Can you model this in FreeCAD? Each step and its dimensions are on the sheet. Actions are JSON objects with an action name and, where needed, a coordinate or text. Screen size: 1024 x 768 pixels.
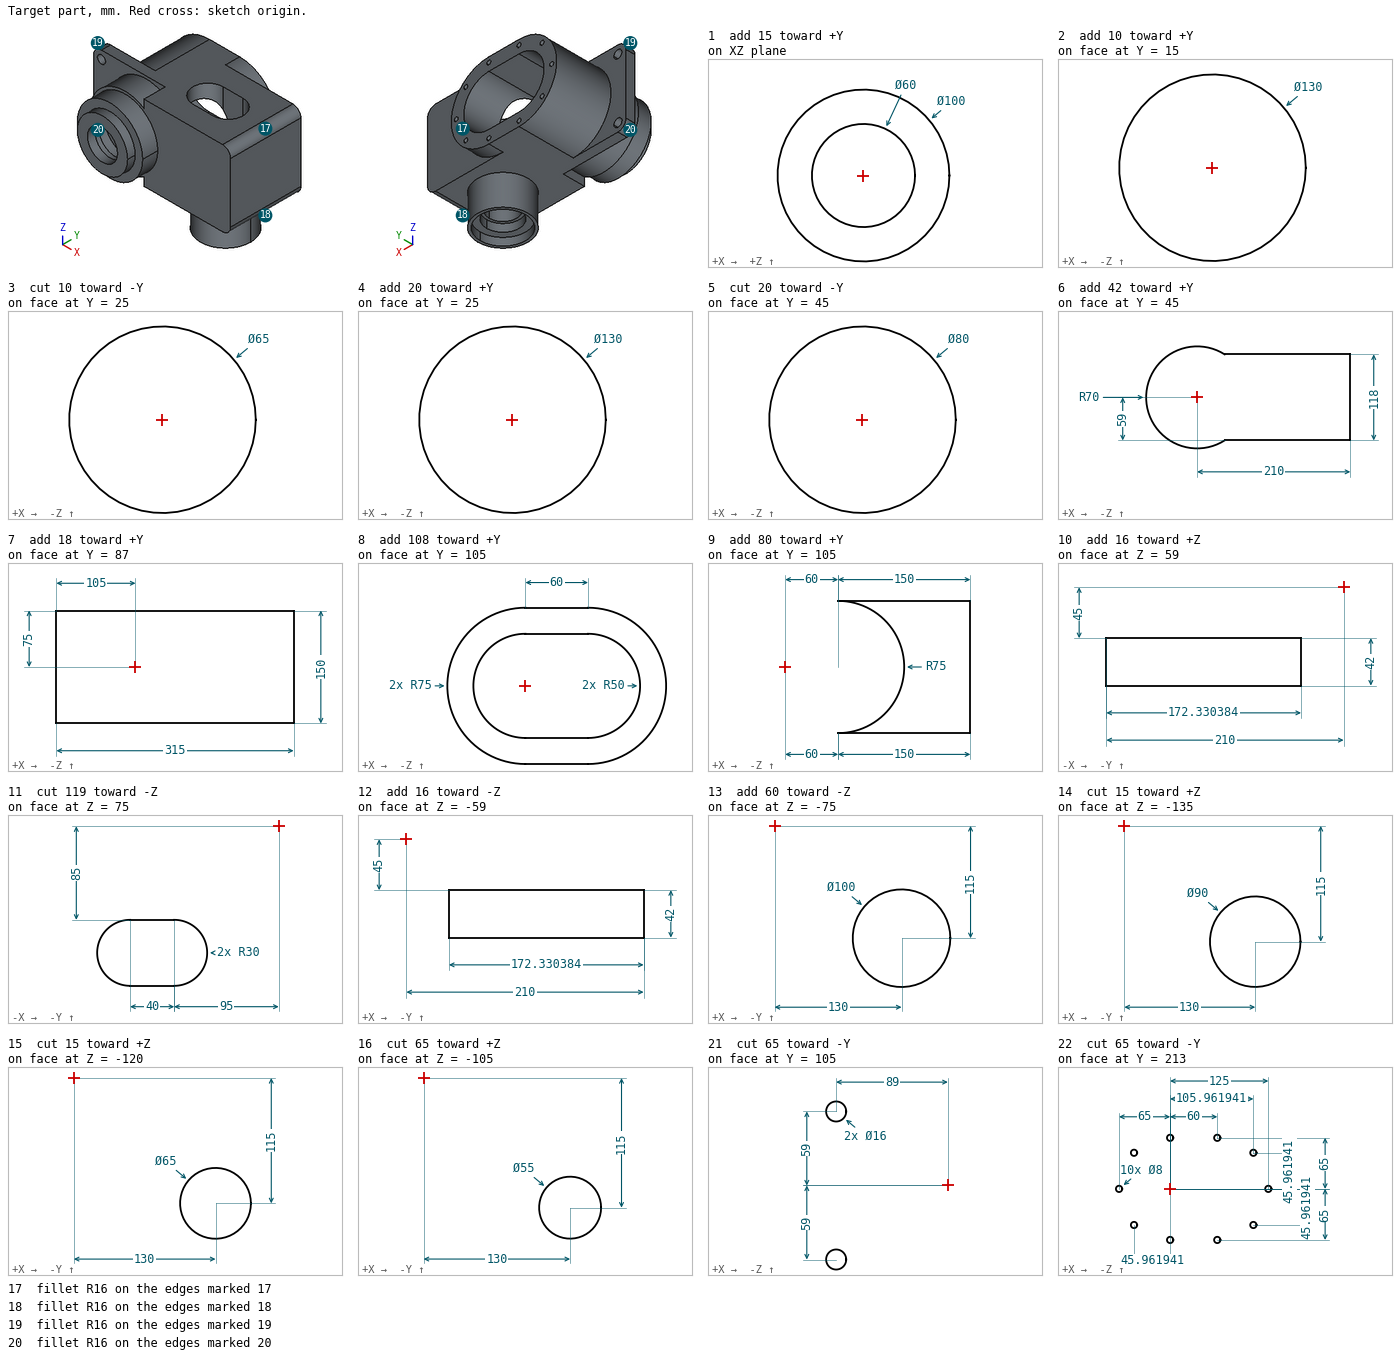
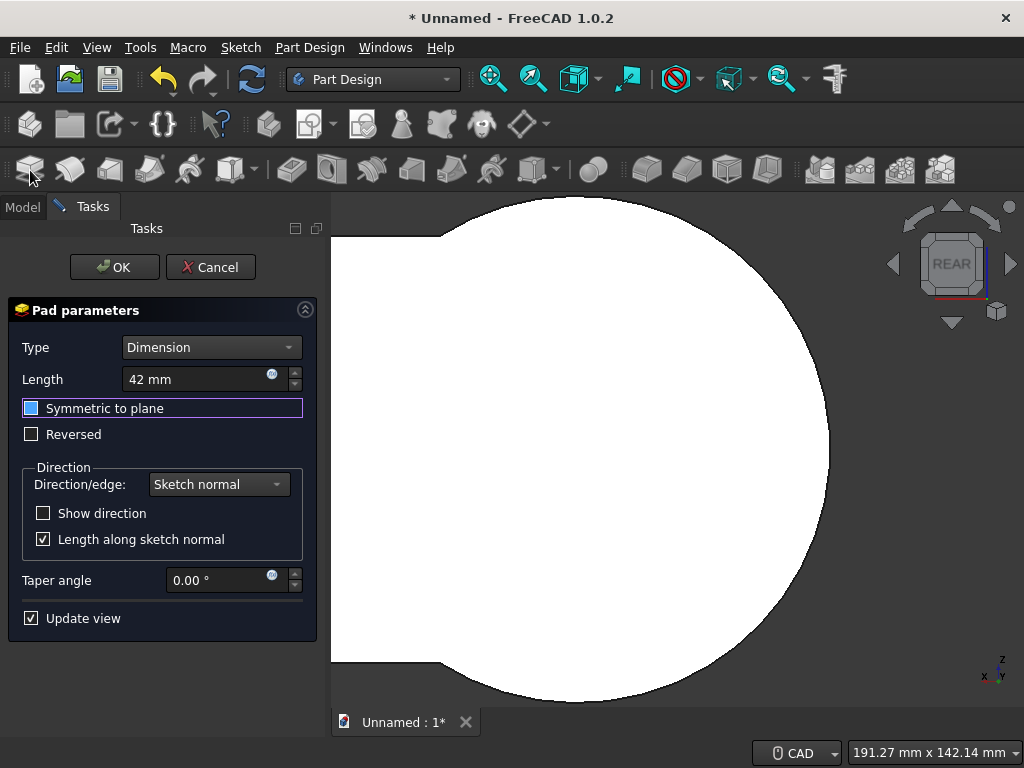
{"action": "left_click", "coordinate": [115, 267]}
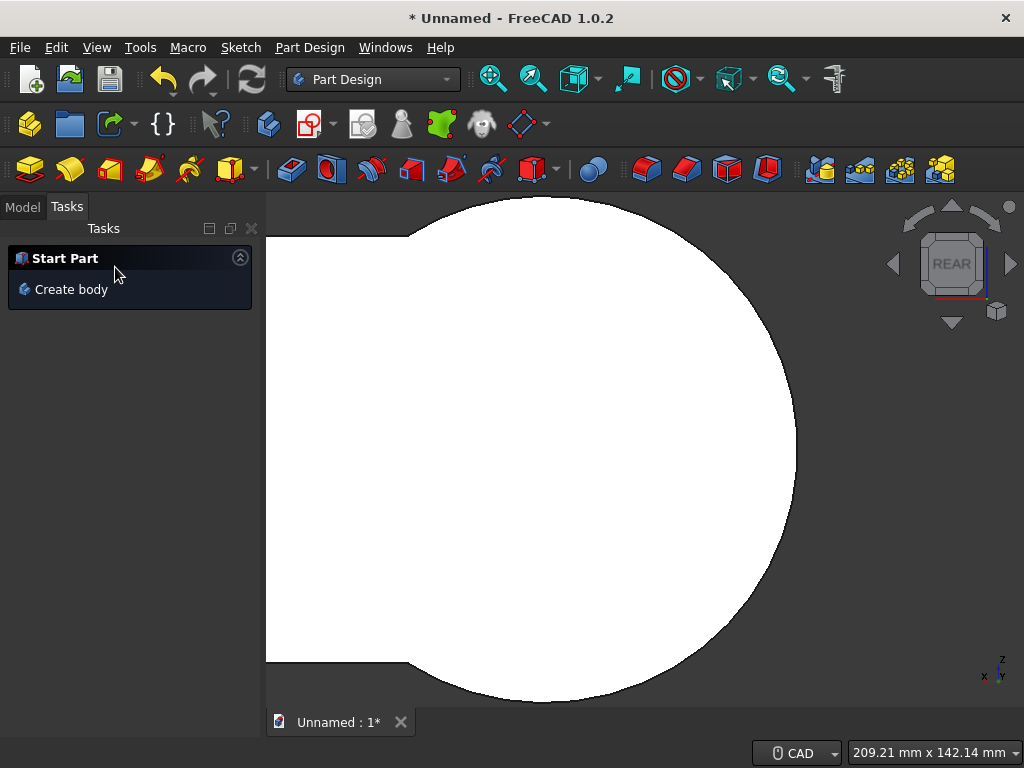
{"action": "left_click", "coordinate": [494, 80]}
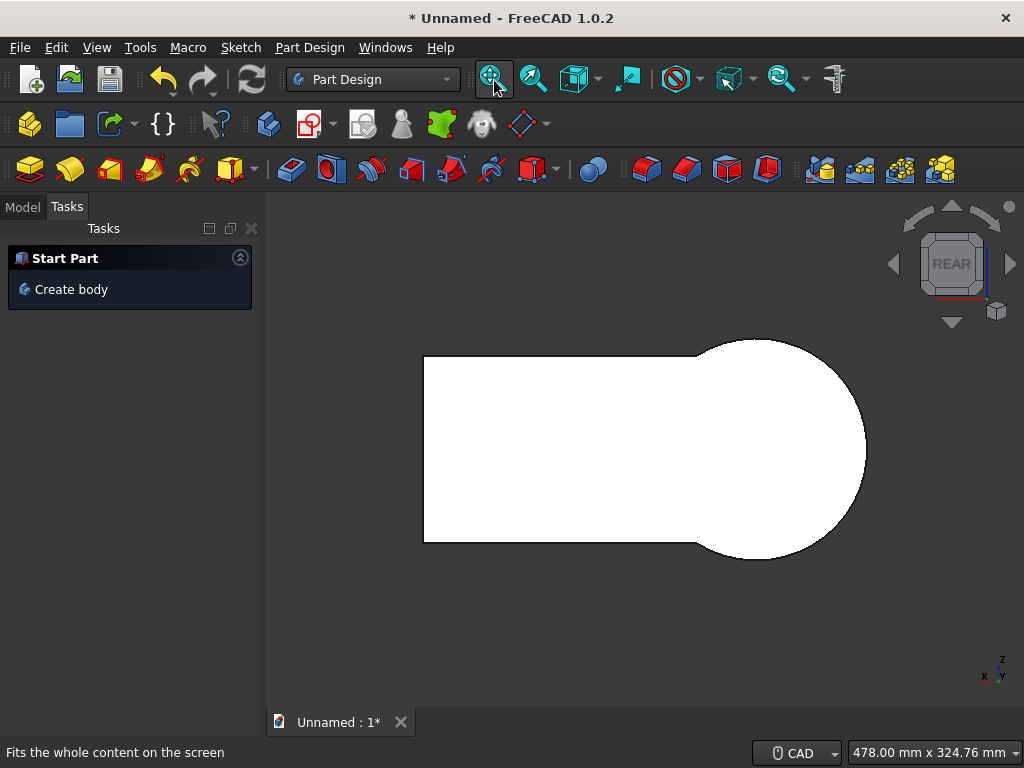
{"action": "left_click", "coordinate": [772, 448]}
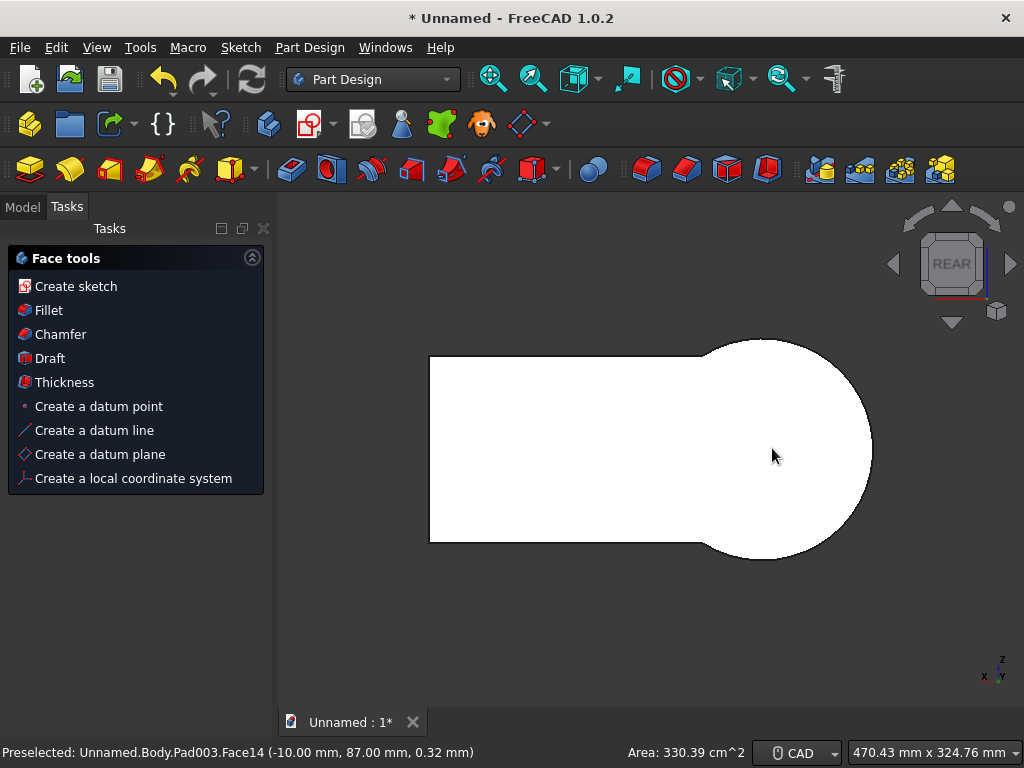
{"action": "left_click", "coordinate": [310, 124]}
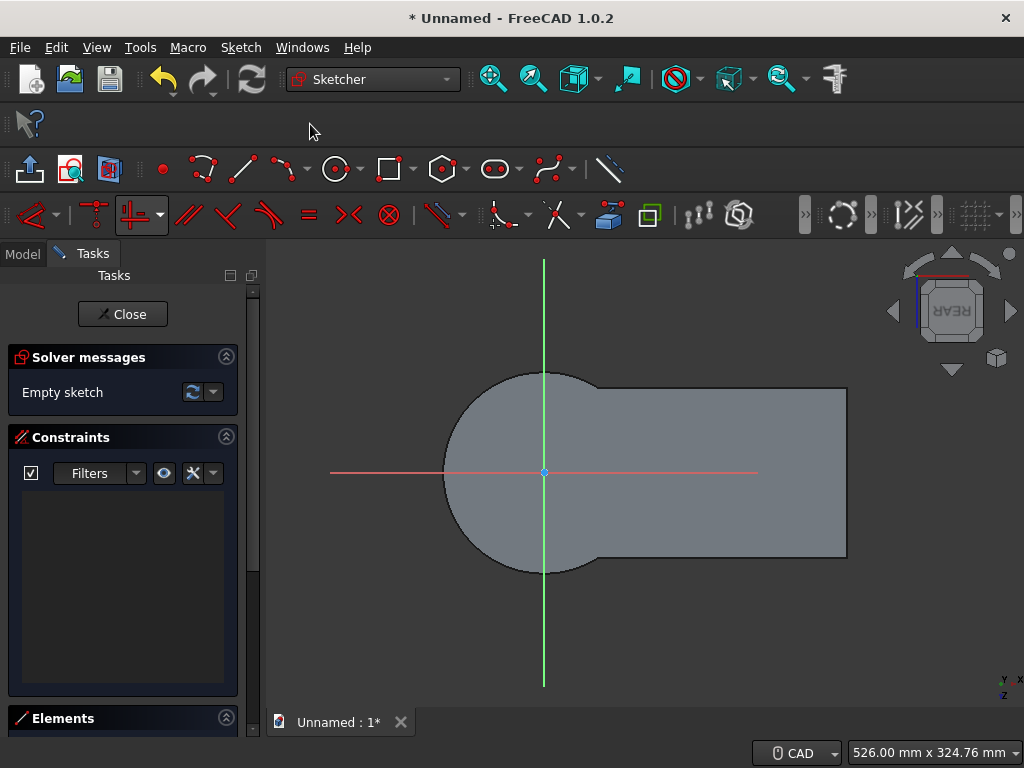
{"action": "scroll", "coordinate": [382, 473], "scroll_direction": "down", "scroll_amount": 1}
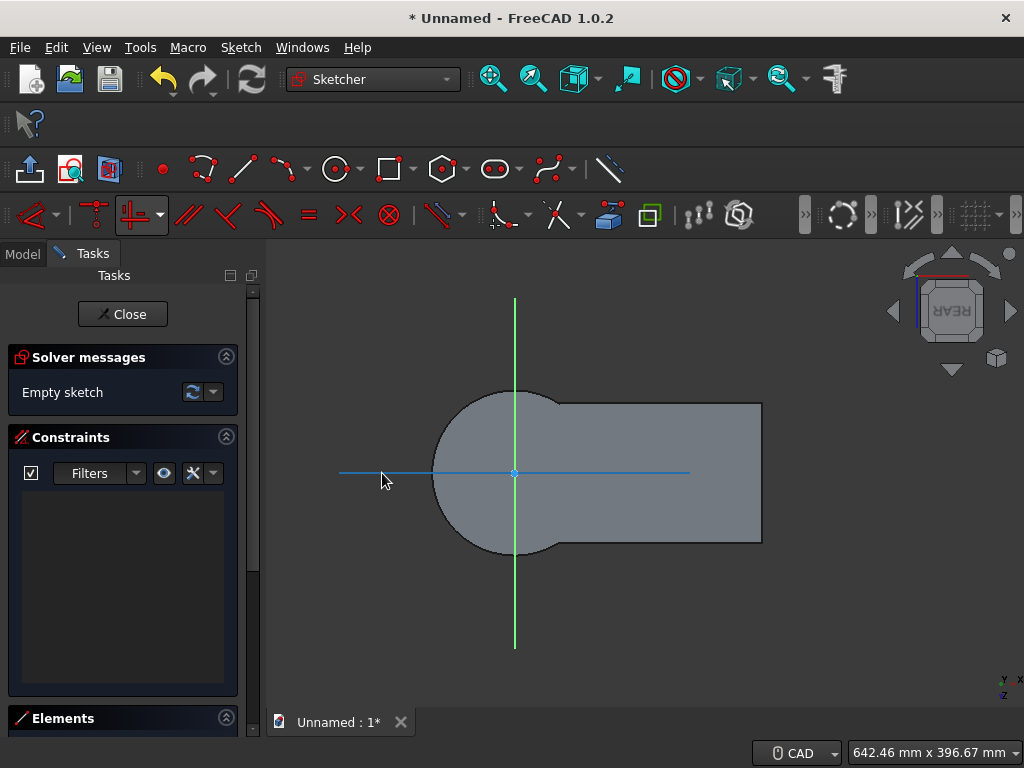
{"action": "left_click", "coordinate": [390, 170]}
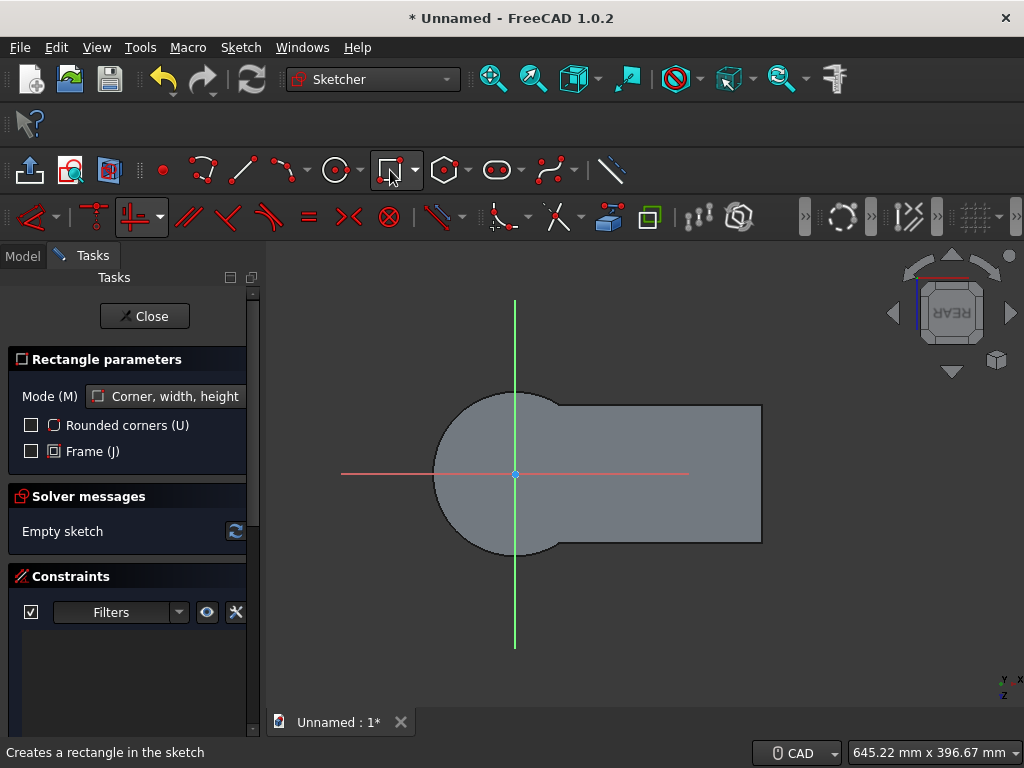
{"action": "left_click", "coordinate": [392, 386]}
{"action": "mouse_move", "coordinate": [762, 562]}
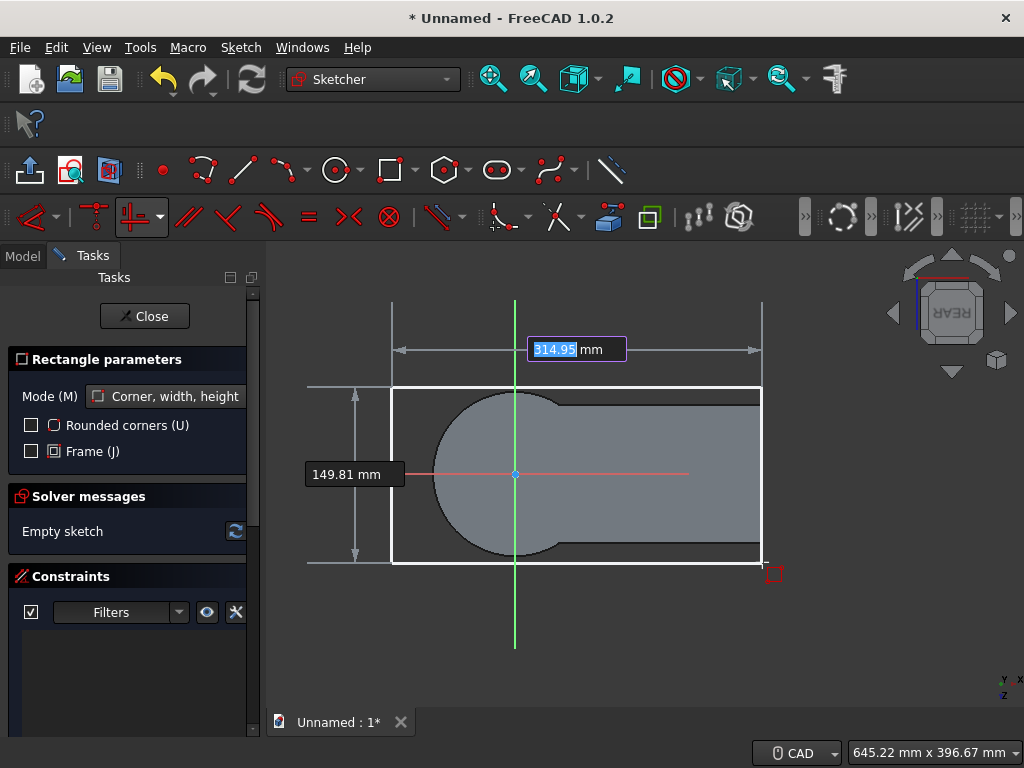
{"action": "type", "text": "315"}
{"action": "key", "text": "Tab"}
{"action": "type", "text": "150"}
{"action": "key", "text": "Return"}
{"action": "key", "text": "Escape"}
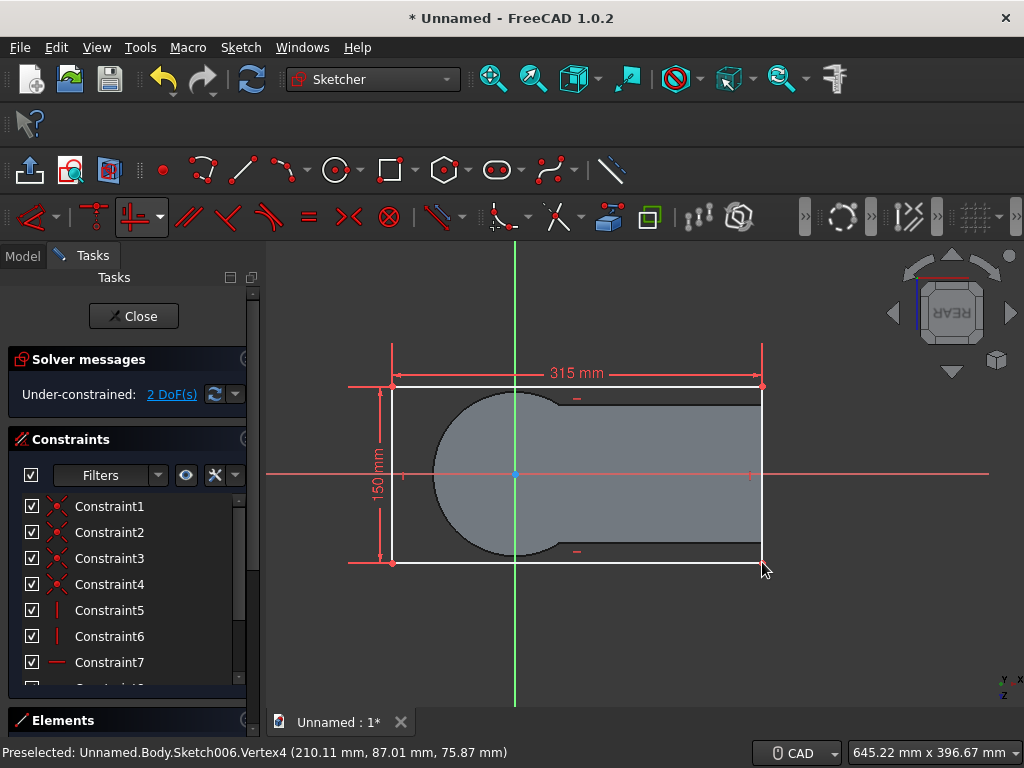
{"action": "left_click", "coordinate": [32, 218]}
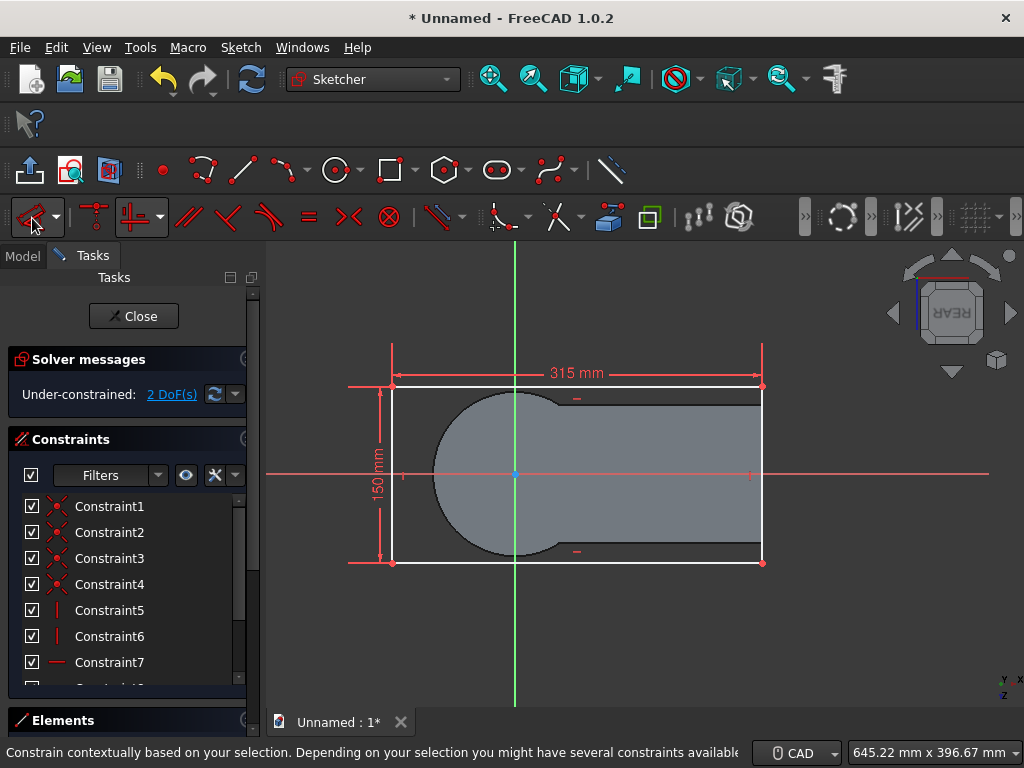
{"action": "left_click", "coordinate": [392, 387]}
{"action": "left_click", "coordinate": [358, 431]}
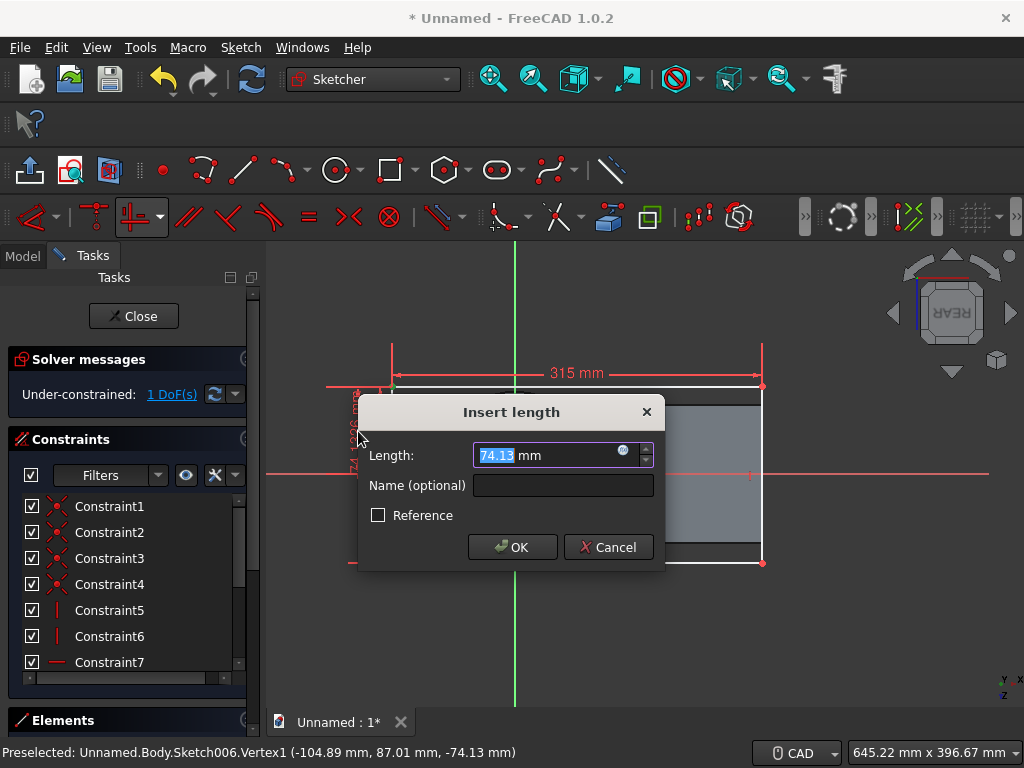
{"action": "type", "text": "75"}
{"action": "key", "text": "Return"}